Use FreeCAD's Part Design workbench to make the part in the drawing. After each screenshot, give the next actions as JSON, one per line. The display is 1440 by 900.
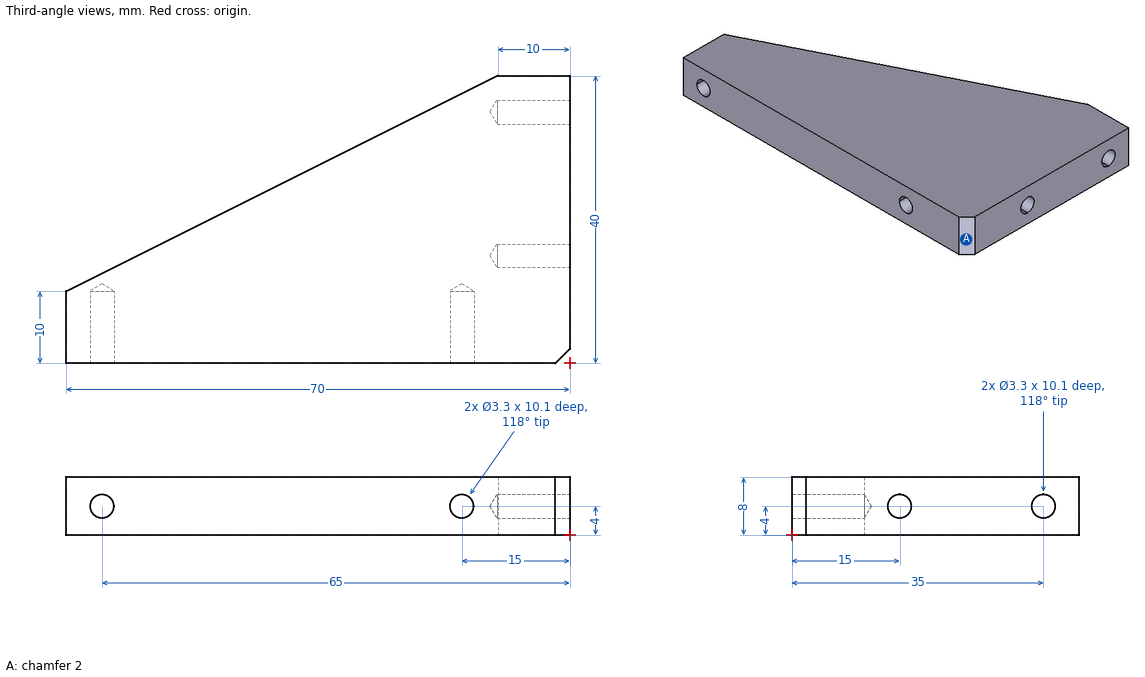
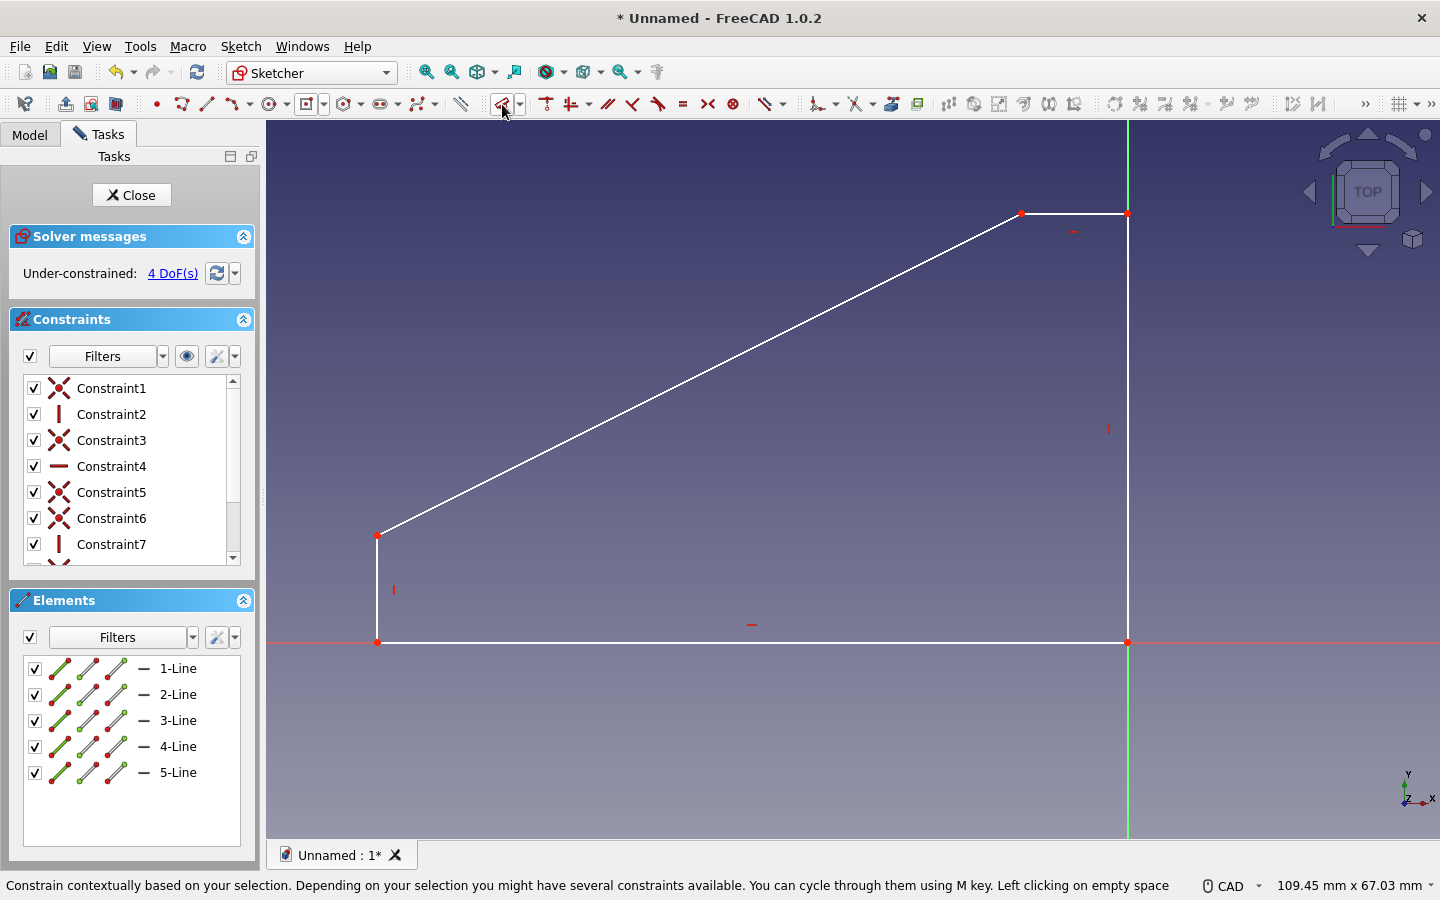
{"action": "left_click", "coordinate": [1128, 514]}
{"action": "left_click", "coordinate": [1162, 428]}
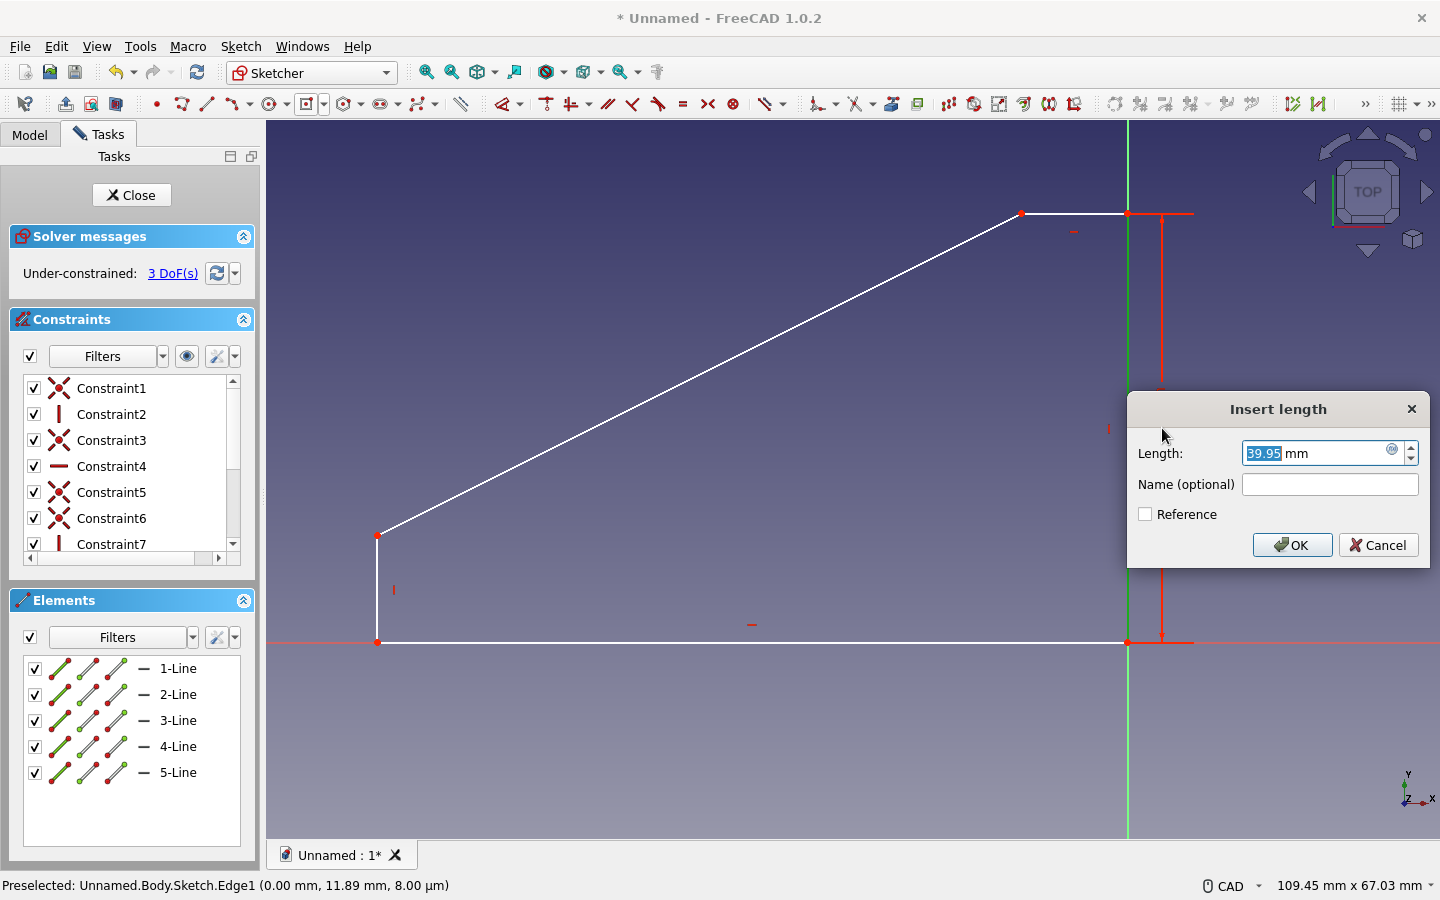
{"action": "type", "text": "40"}
{"action": "key", "text": "Return"}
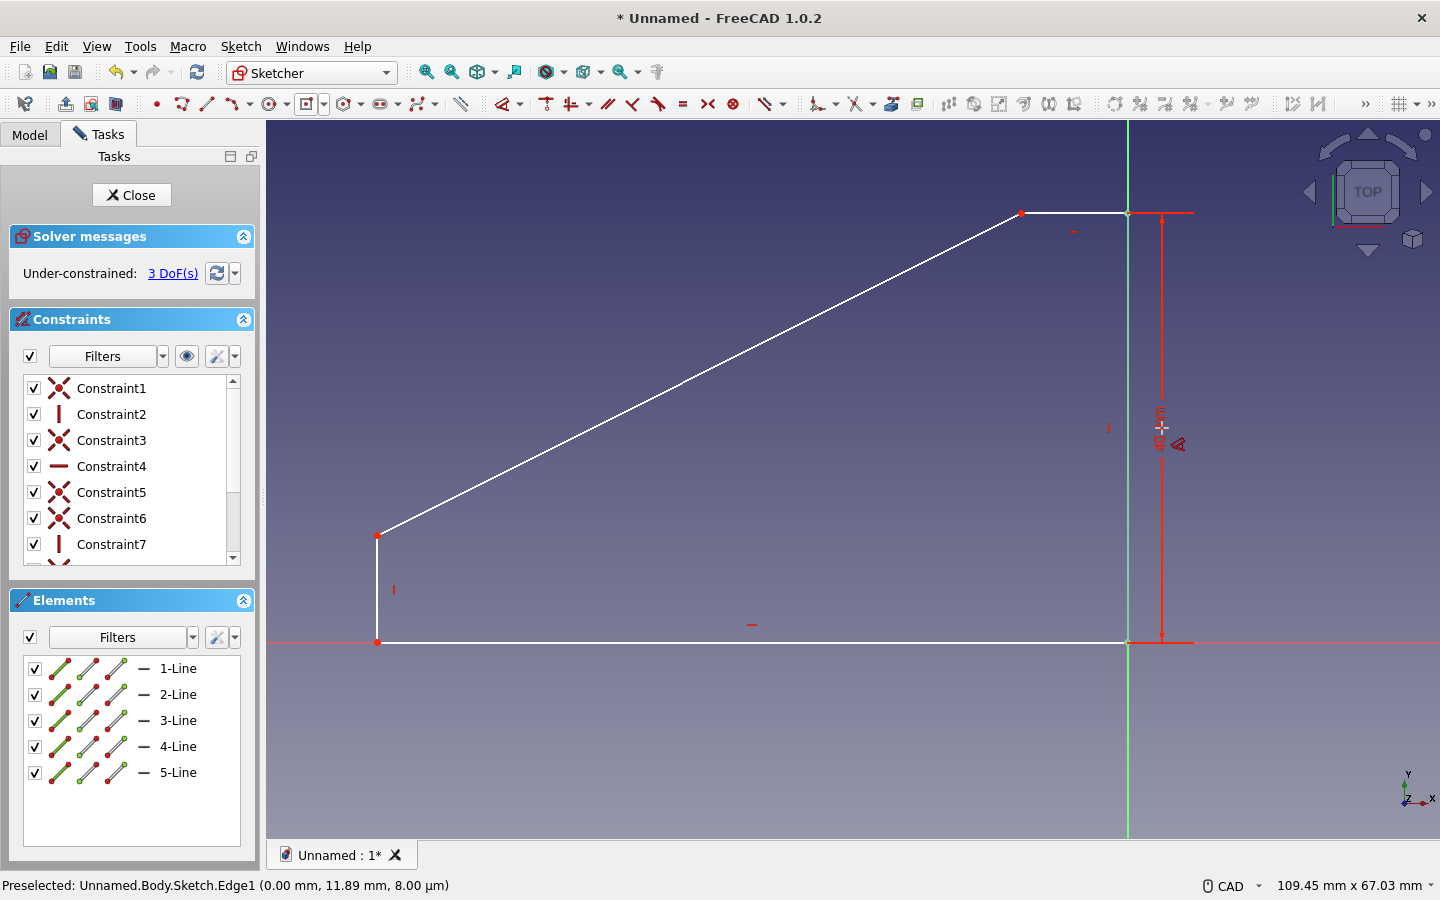
{"action": "left_click", "coordinate": [1096, 213]}
{"action": "left_click", "coordinate": [1074, 179]}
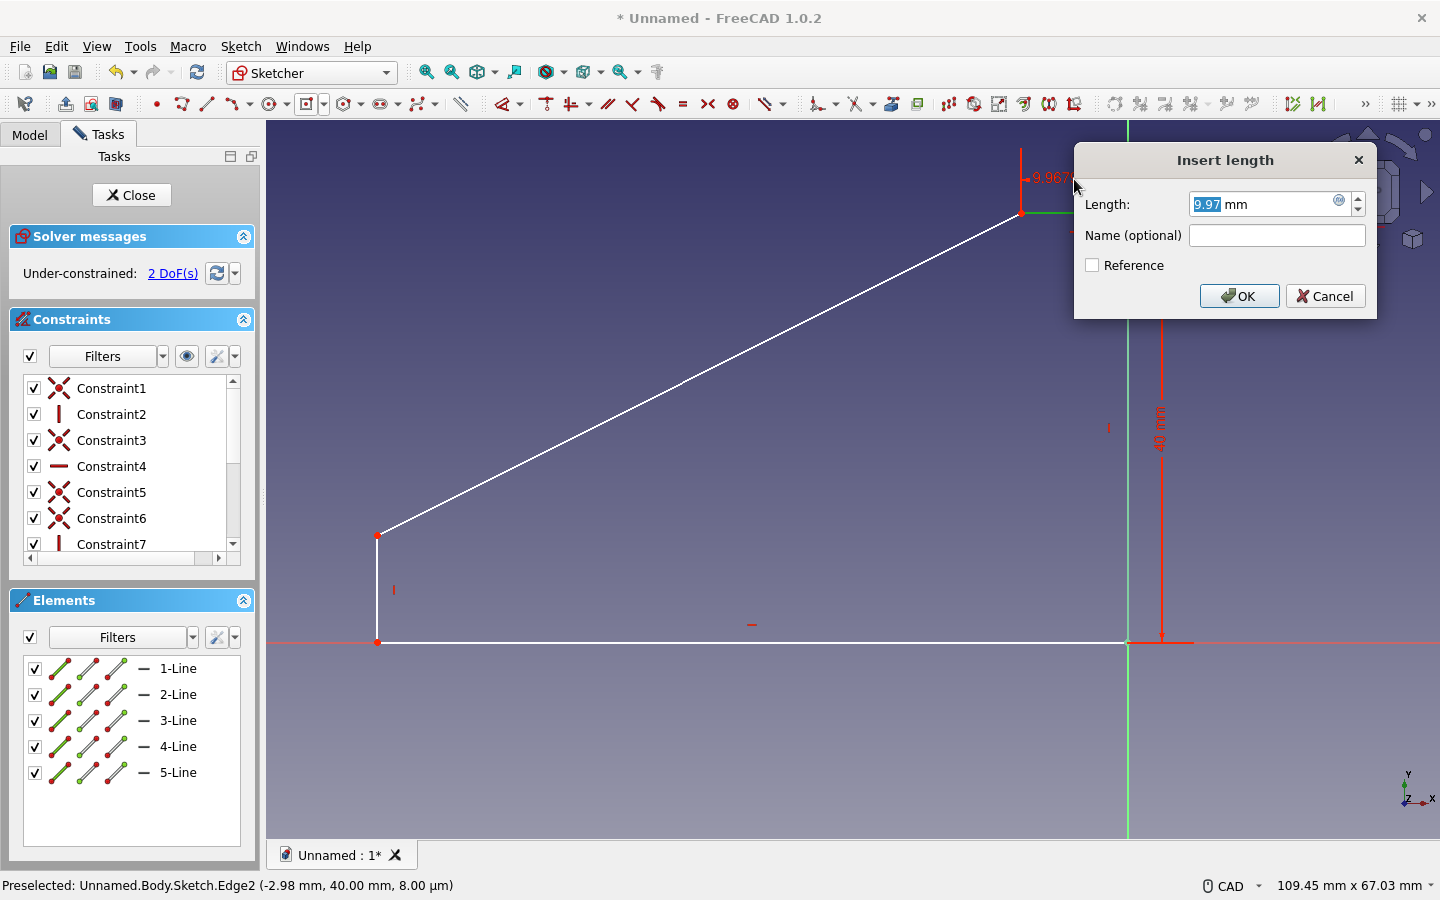
{"action": "type", "text": "10"}
{"action": "key", "text": "Return"}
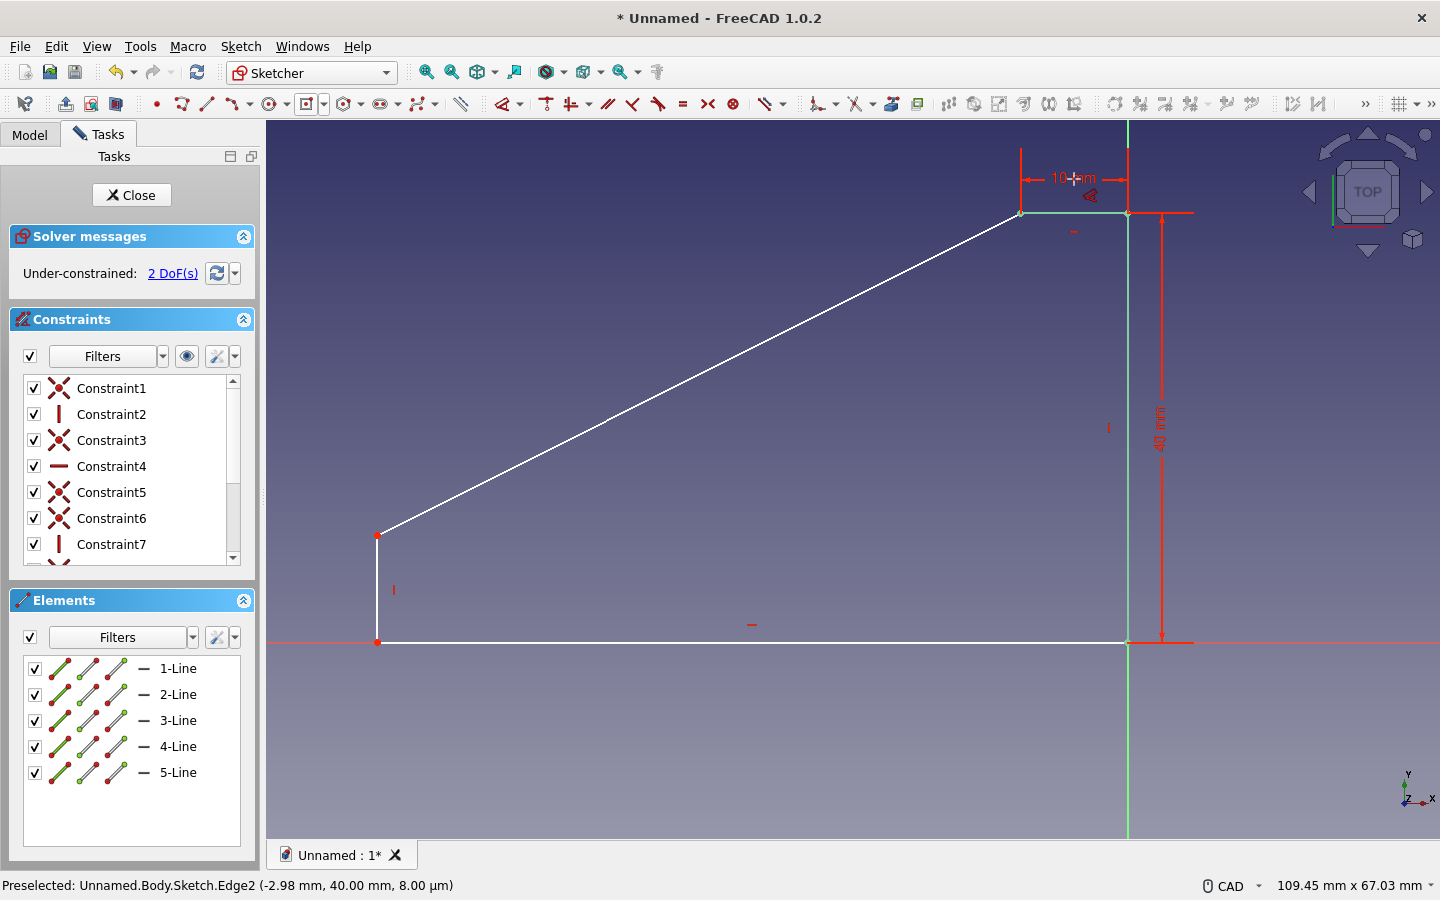
{"action": "left_click", "coordinate": [377, 568]}
{"action": "left_click", "coordinate": [343, 589]}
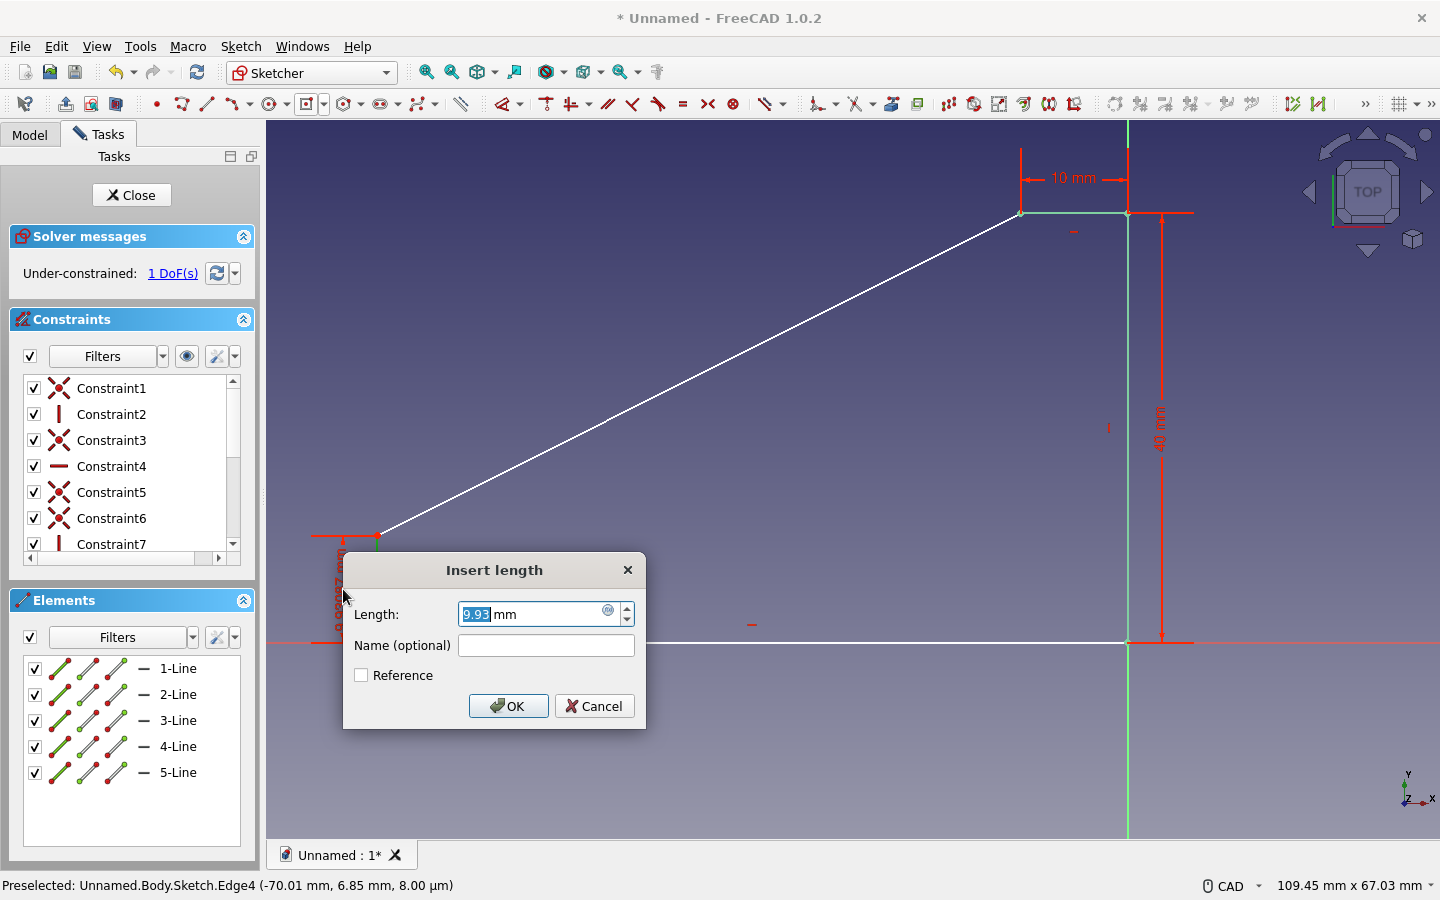
{"action": "type", "text": "10"}
{"action": "key", "text": "Return"}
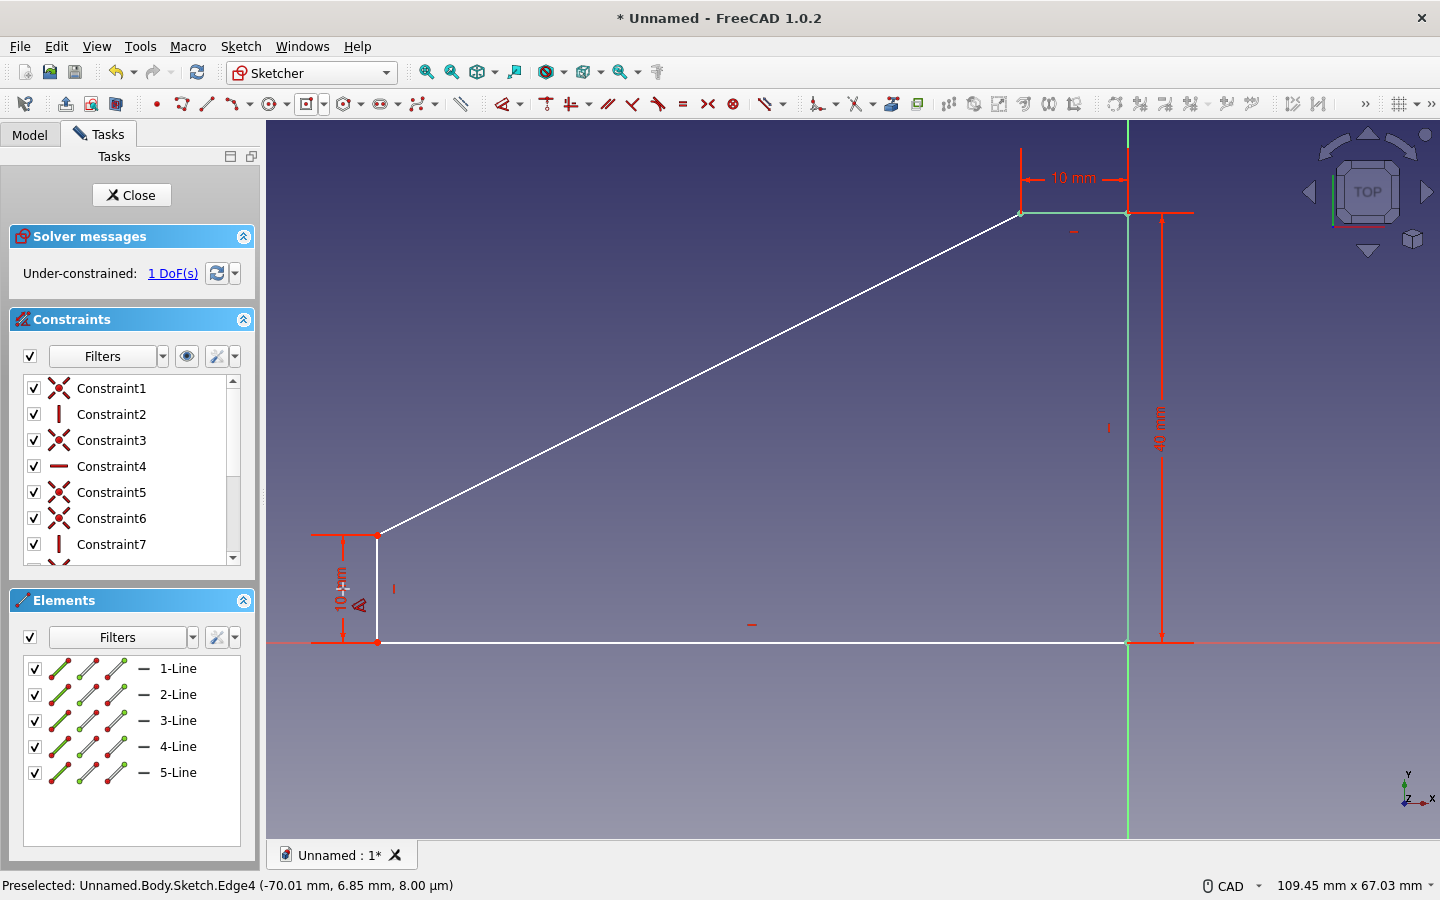
{"action": "left_click", "coordinate": [602, 643]}
{"action": "left_click", "coordinate": [752, 677]}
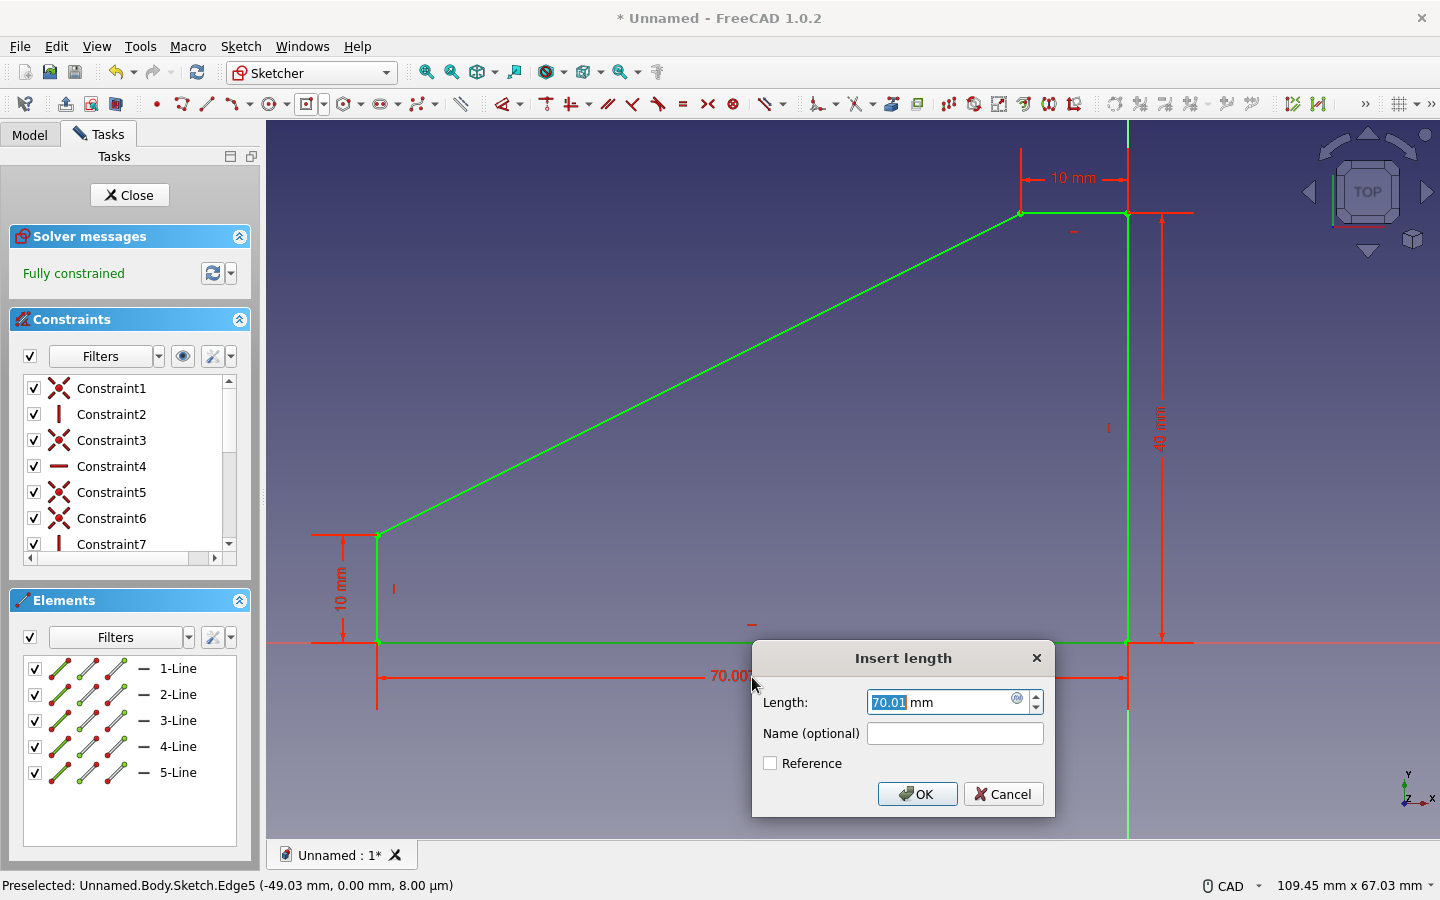
{"action": "type", "text": "70"}
{"action": "key", "text": "Return"}
{"action": "key", "text": "Escape"}